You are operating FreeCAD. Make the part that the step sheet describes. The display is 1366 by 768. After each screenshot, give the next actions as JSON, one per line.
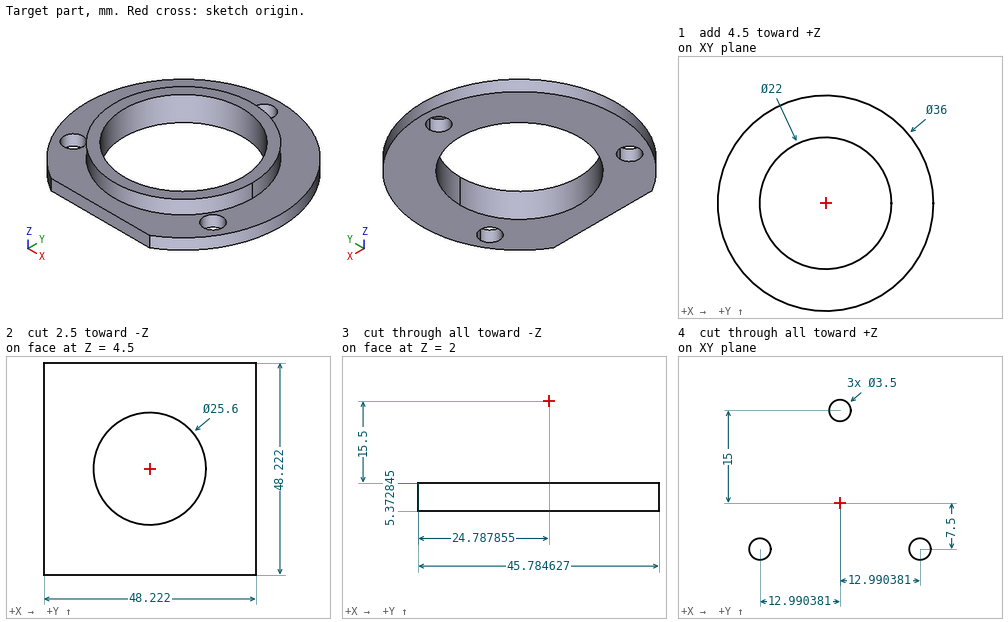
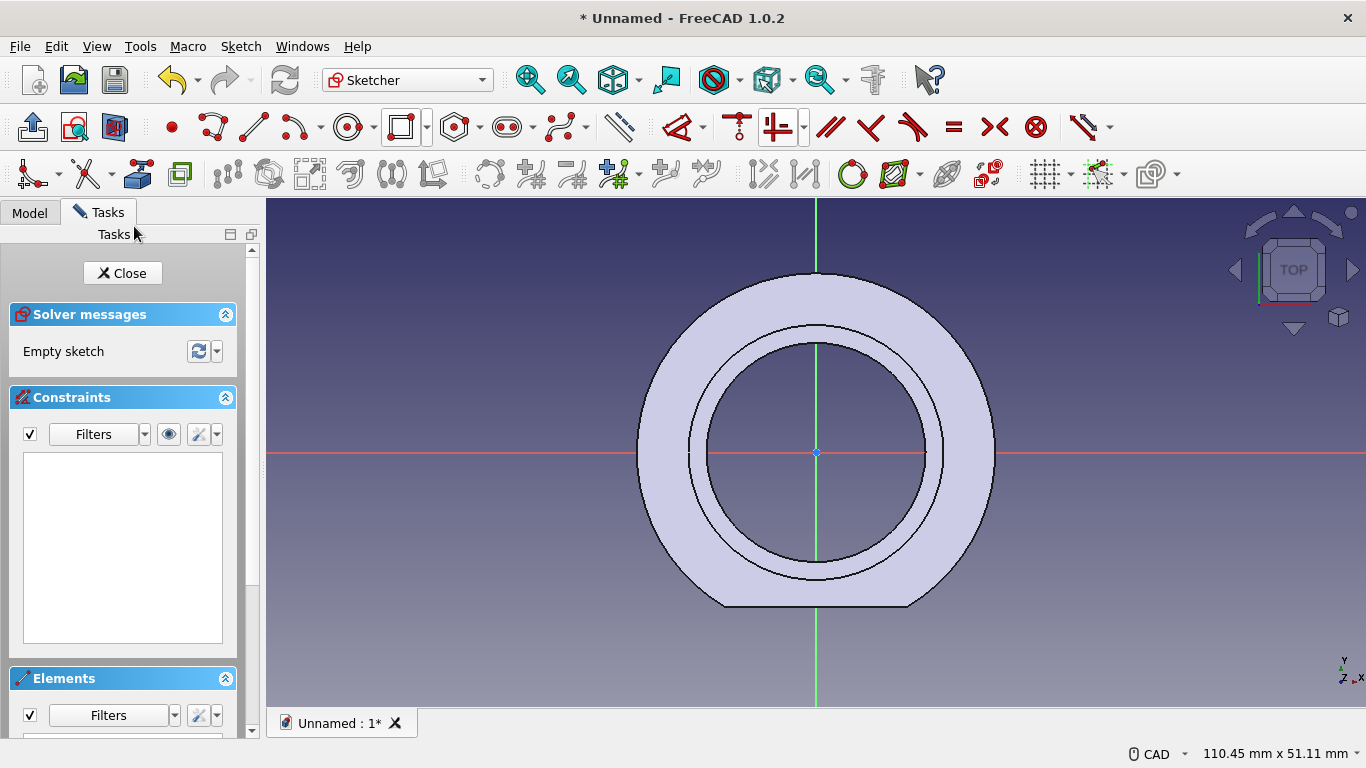
{"action": "left_click", "coordinate": [115, 128]}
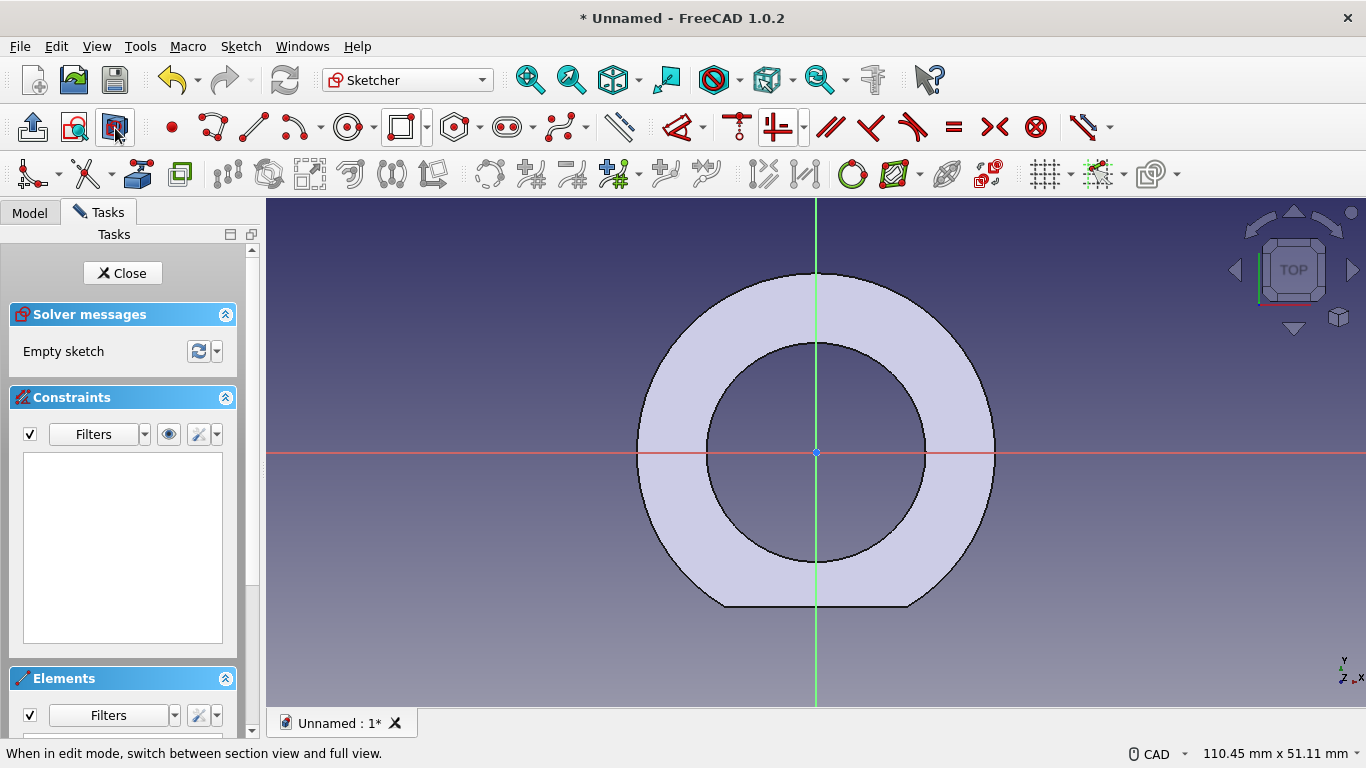
{"action": "left_click", "coordinate": [348, 128]}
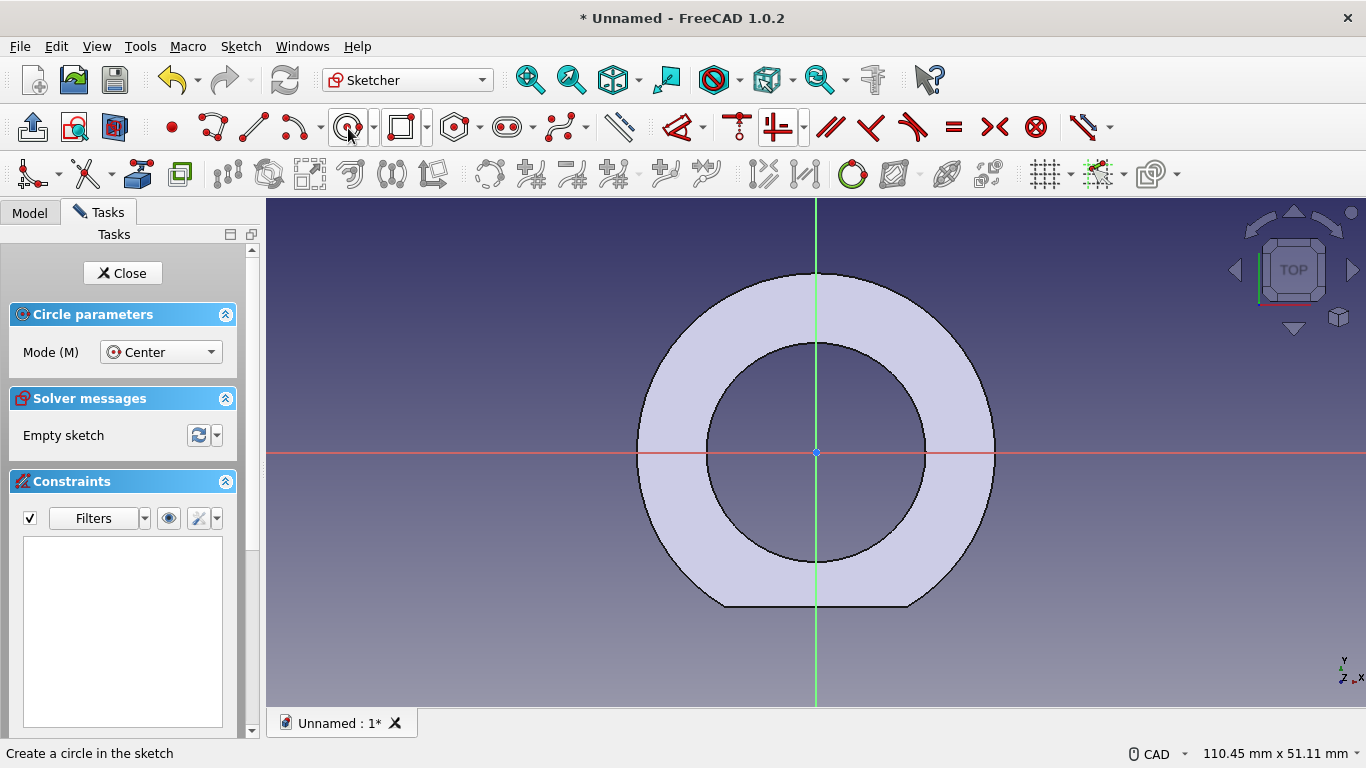
{"action": "scroll", "coordinate": [816, 303], "scroll_direction": "up", "scroll_amount": 2}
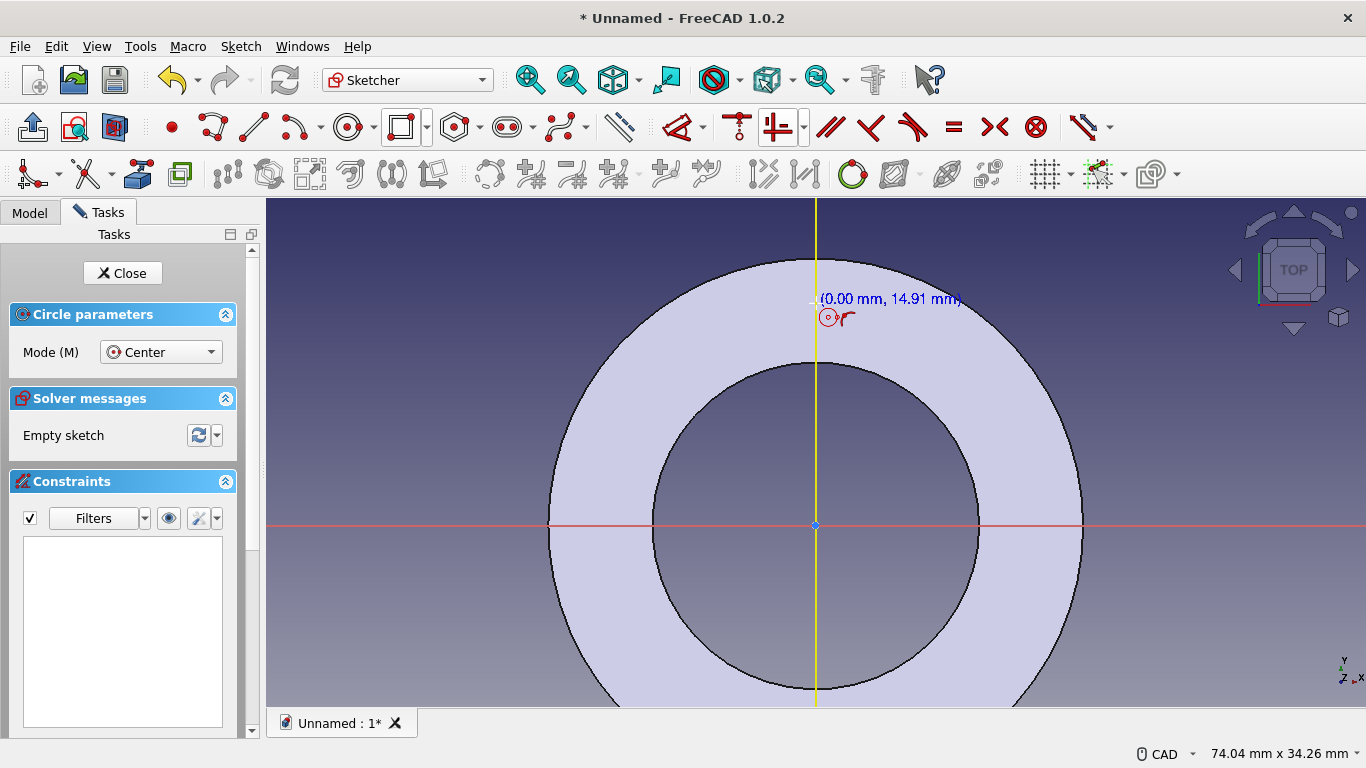
{"action": "left_click", "coordinate": [816, 303]}
{"action": "left_click", "coordinate": [834, 285]}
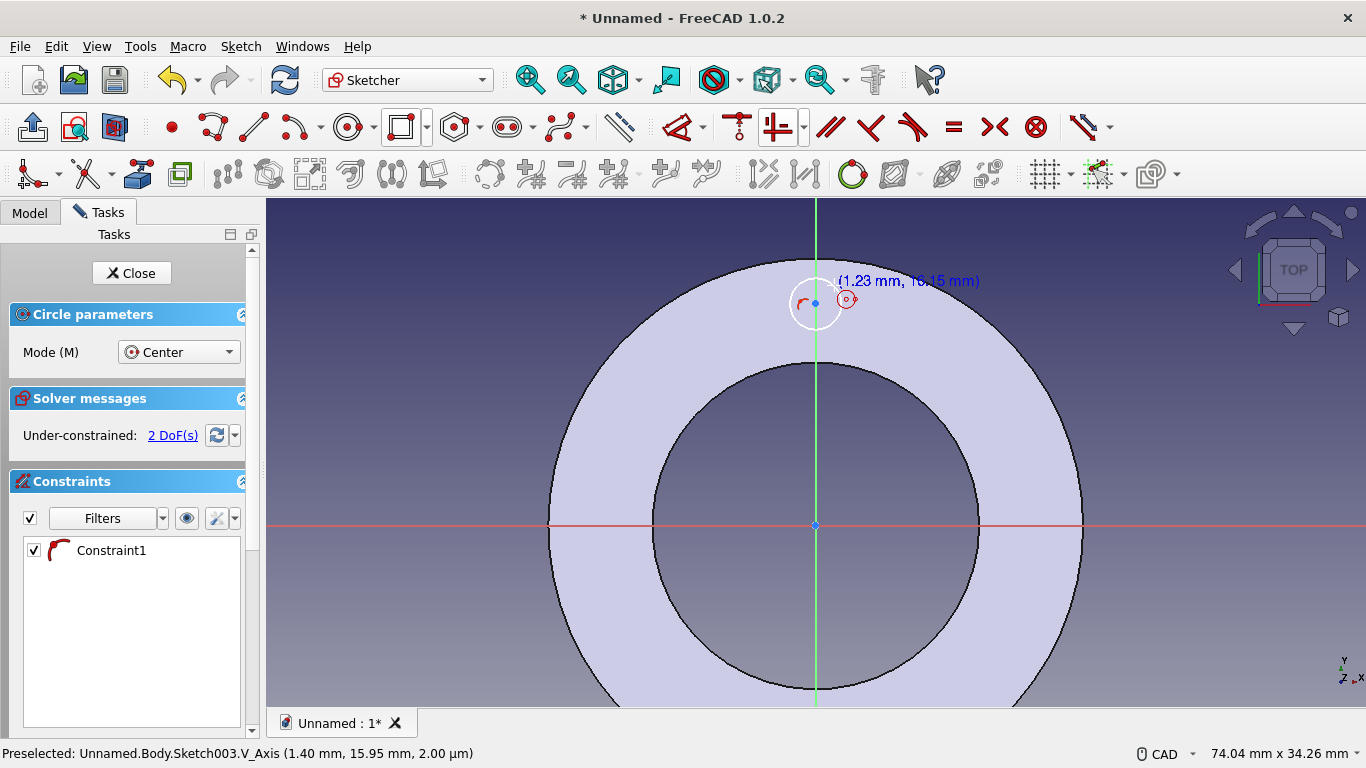
{"action": "left_click", "coordinate": [1009, 637]}
{"action": "left_click", "coordinate": [1027, 619]}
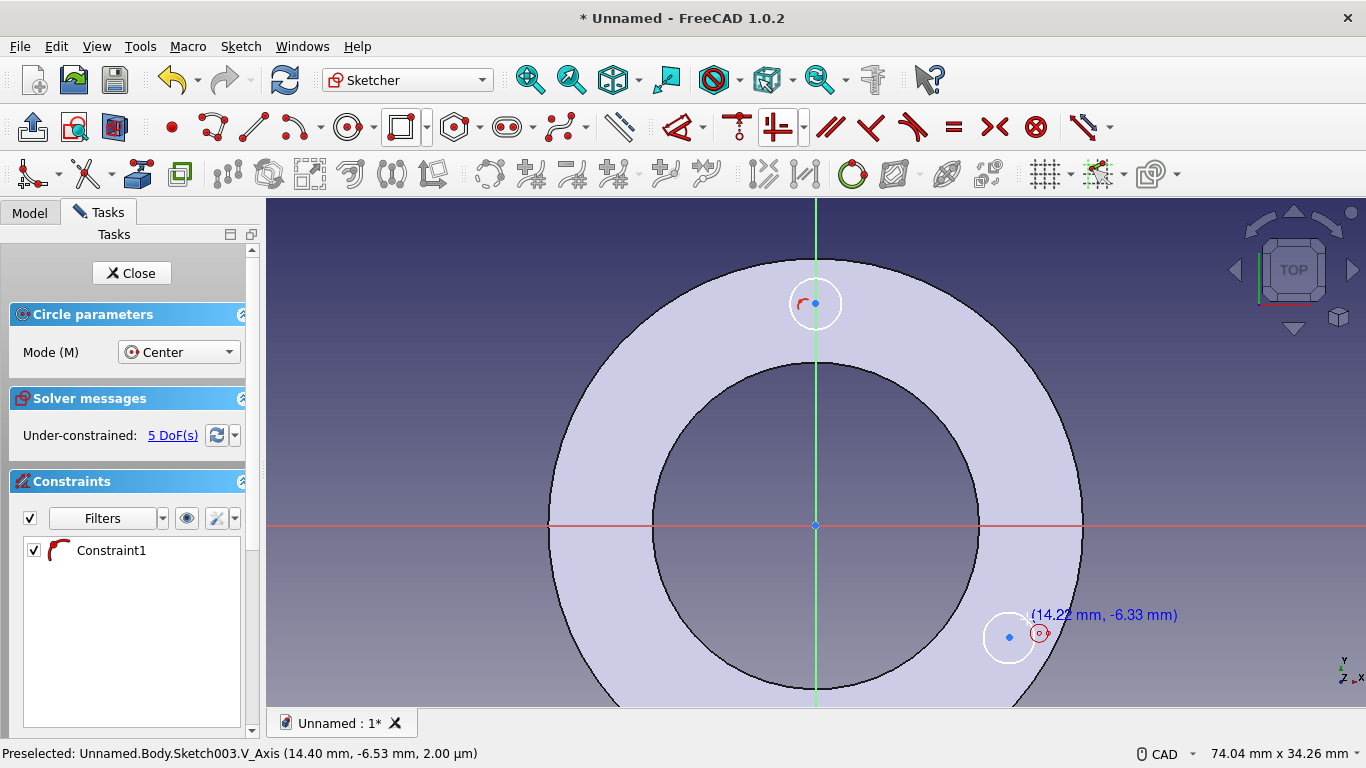
{"action": "left_click", "coordinate": [623, 637]}
{"action": "left_click", "coordinate": [641, 619]}
{"action": "key", "text": "Escape"}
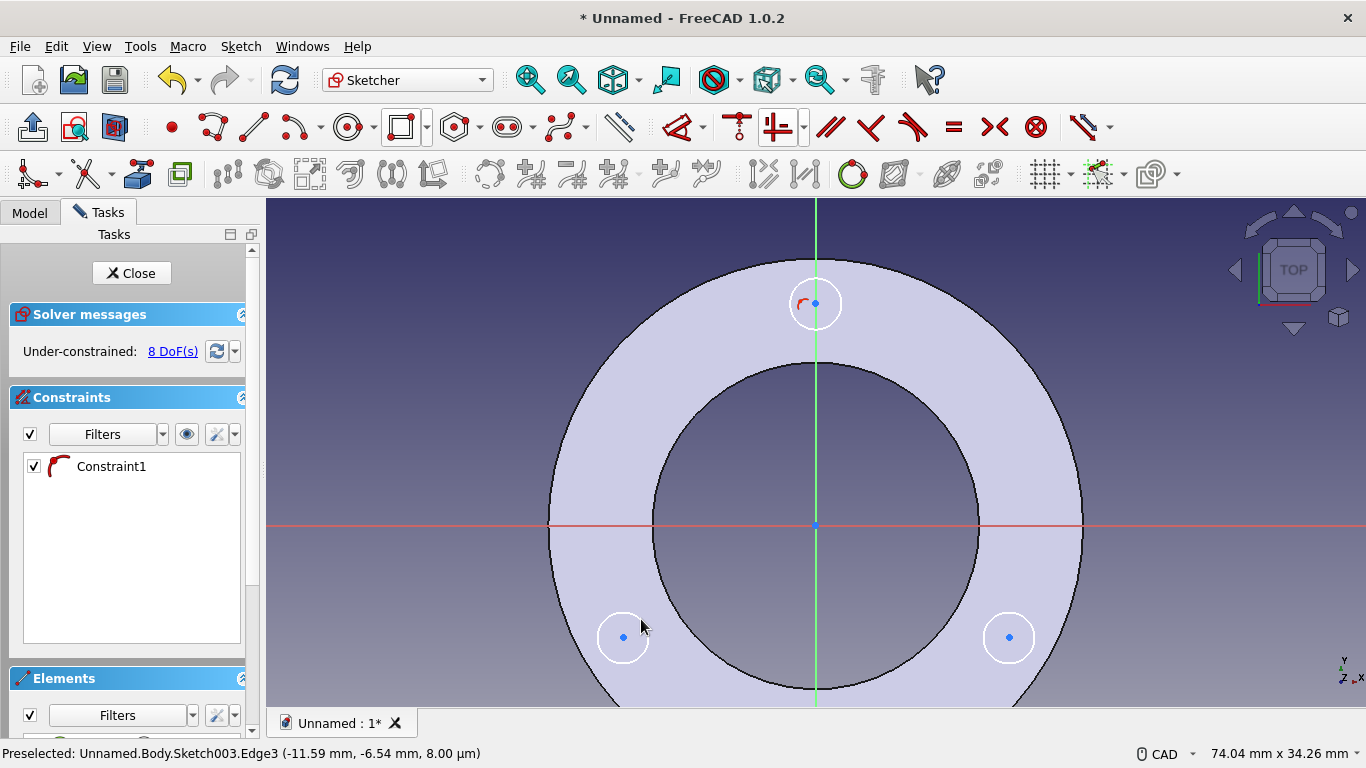
{"action": "left_click", "coordinate": [834, 286]}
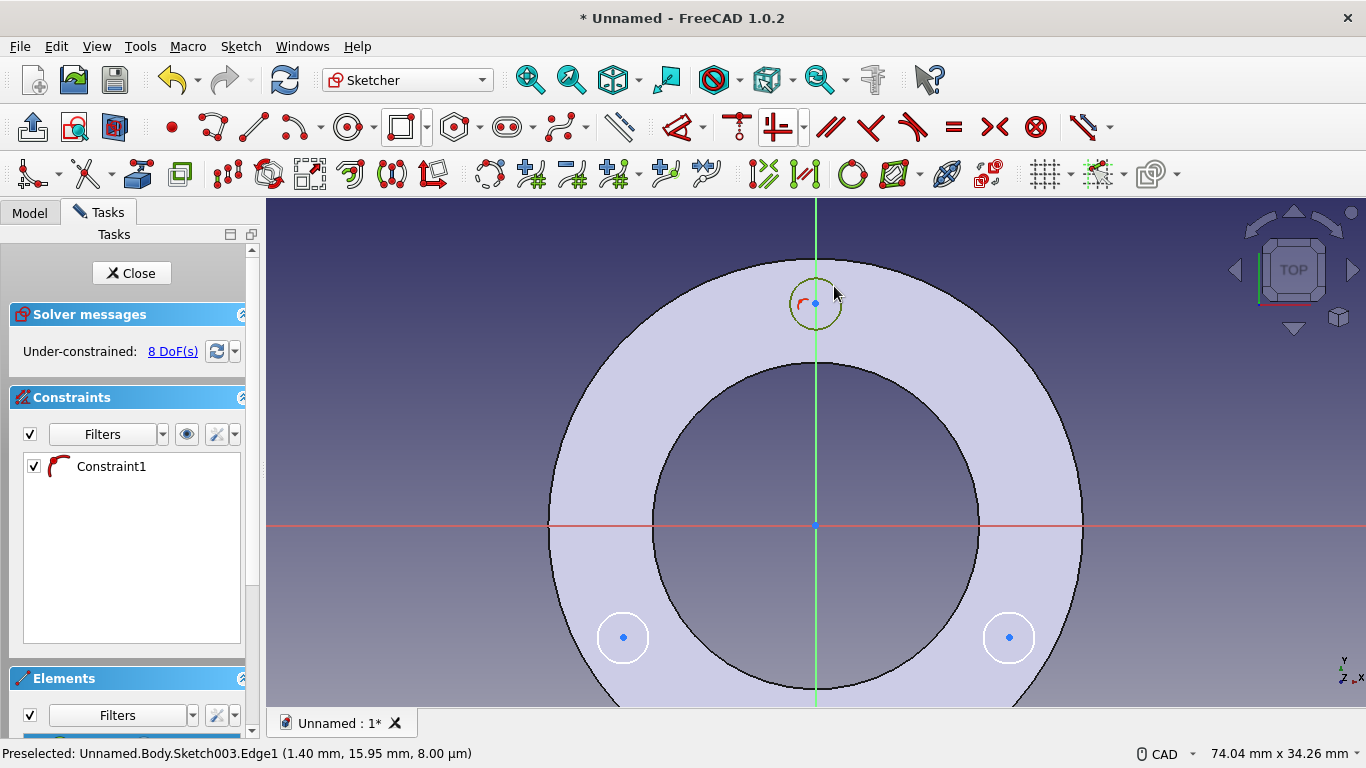
{"action": "left_click", "coordinate": [1027, 620]}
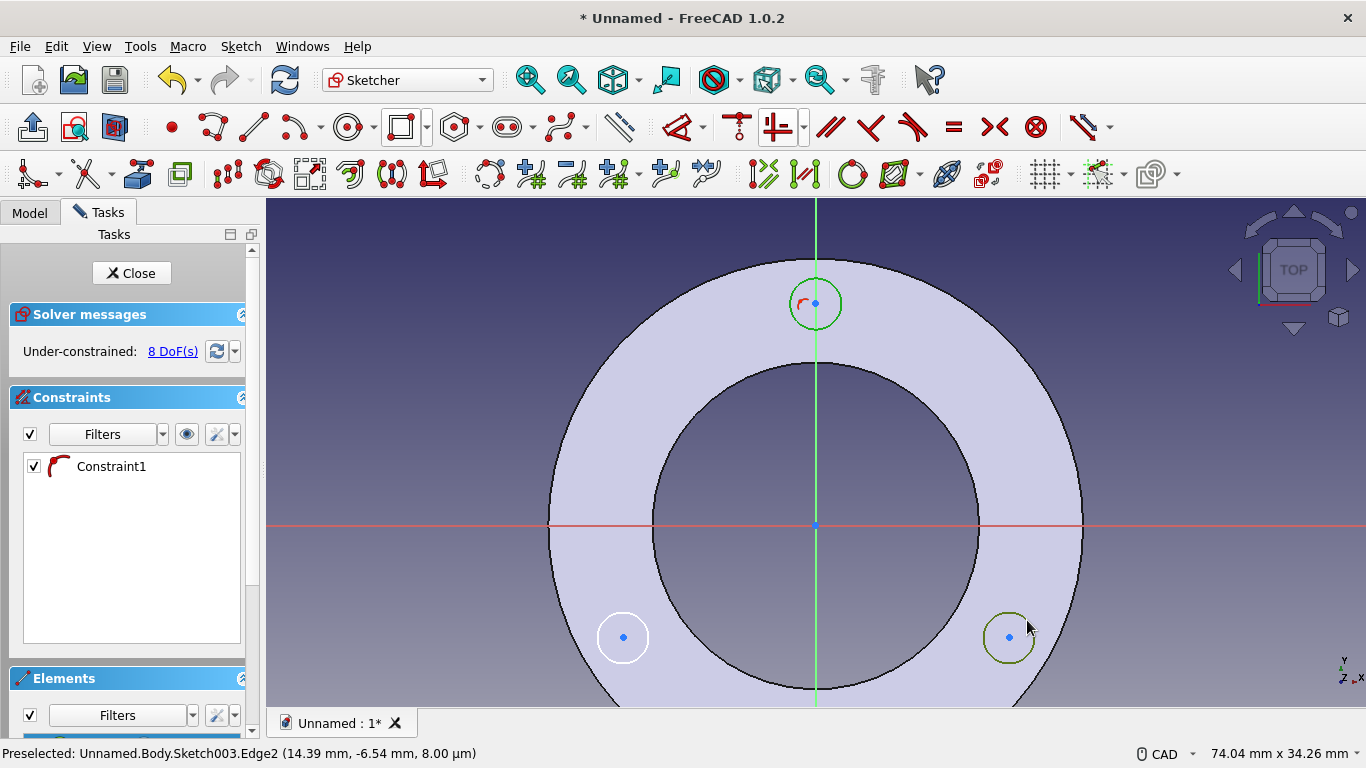
{"action": "left_click", "coordinate": [641, 620]}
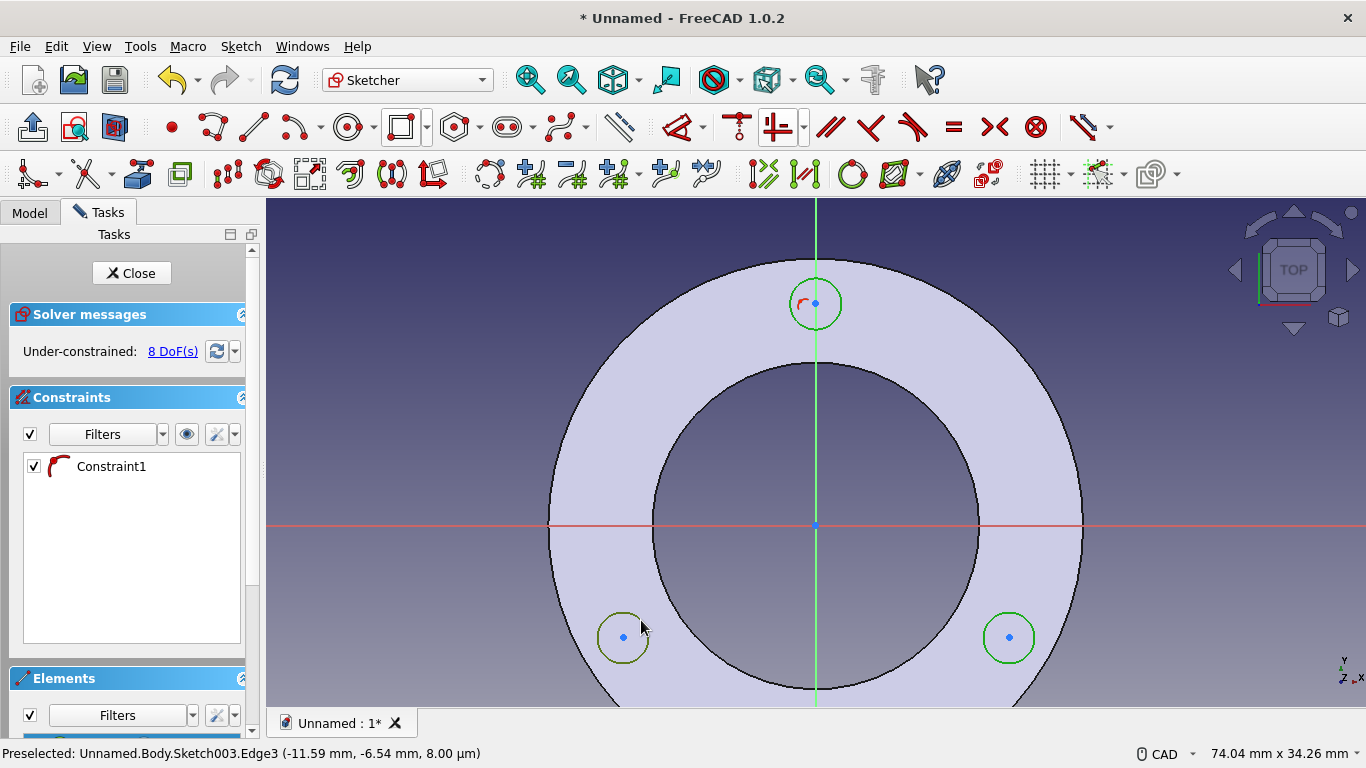
{"action": "left_click", "coordinate": [954, 128]}